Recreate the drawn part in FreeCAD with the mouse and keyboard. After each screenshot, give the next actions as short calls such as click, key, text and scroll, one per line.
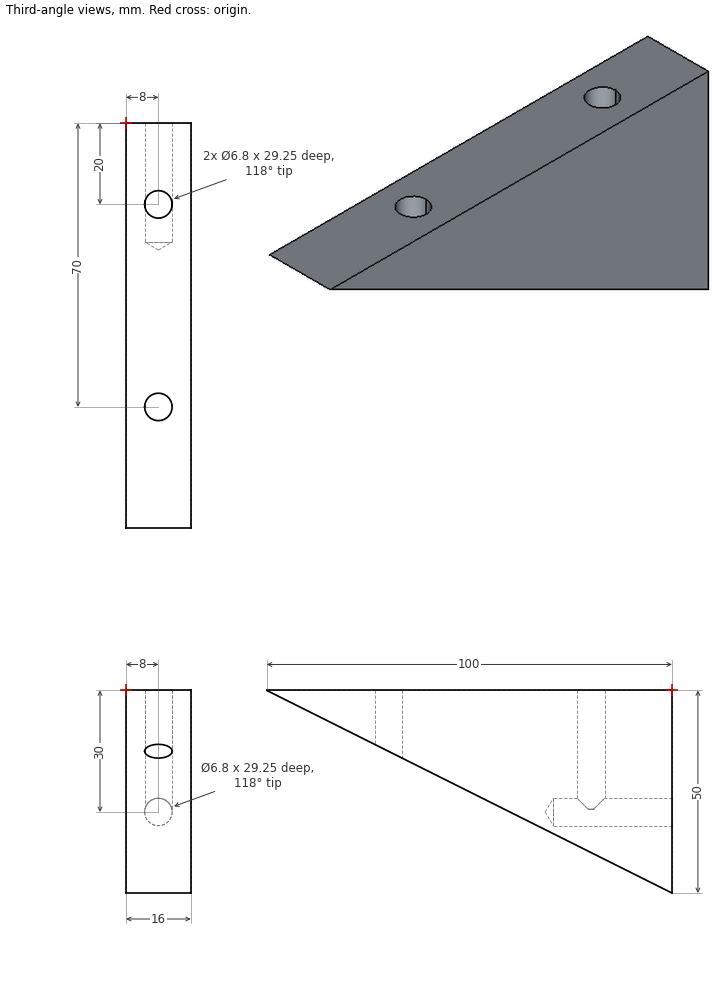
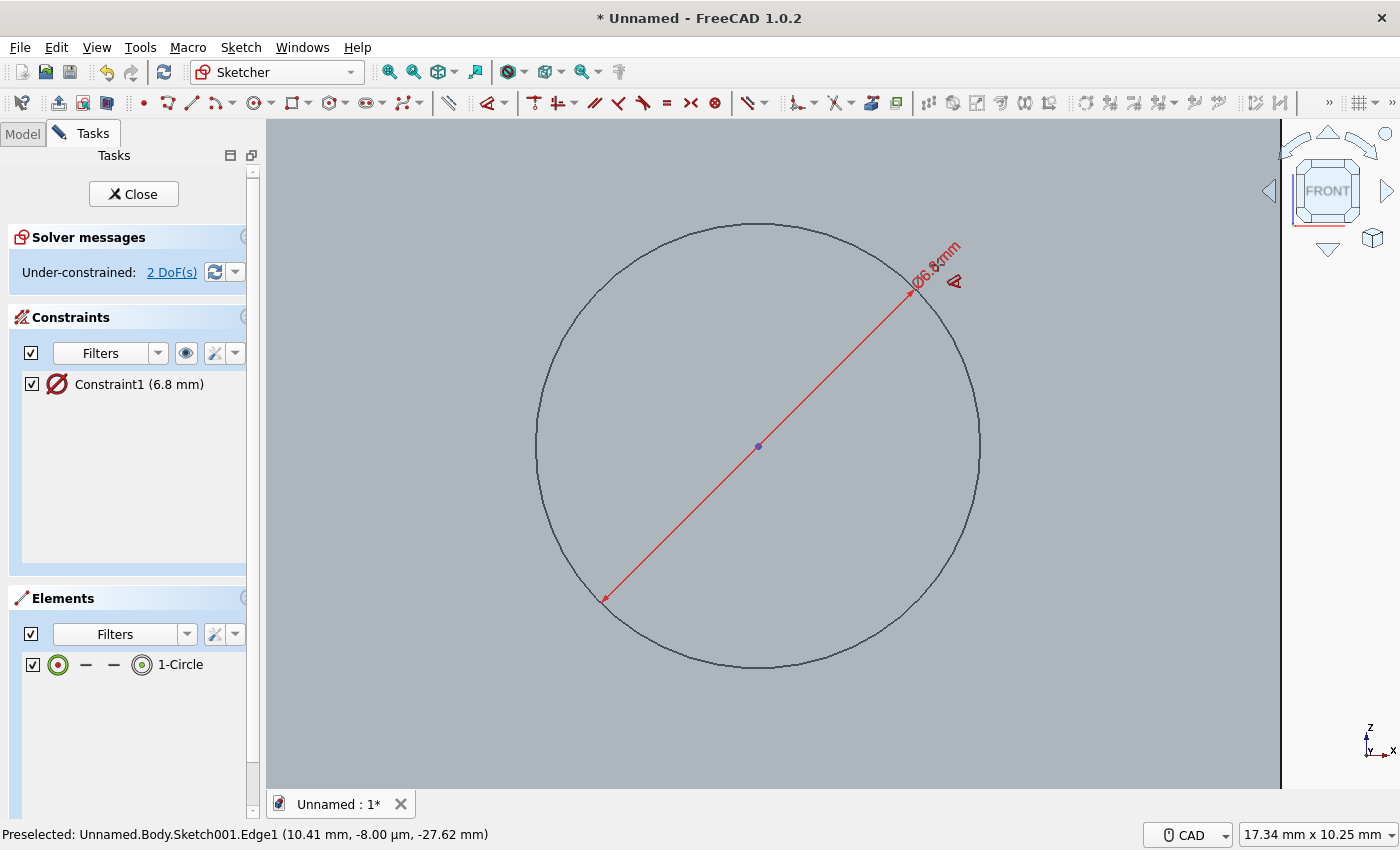
click(758, 446)
click(419, 480)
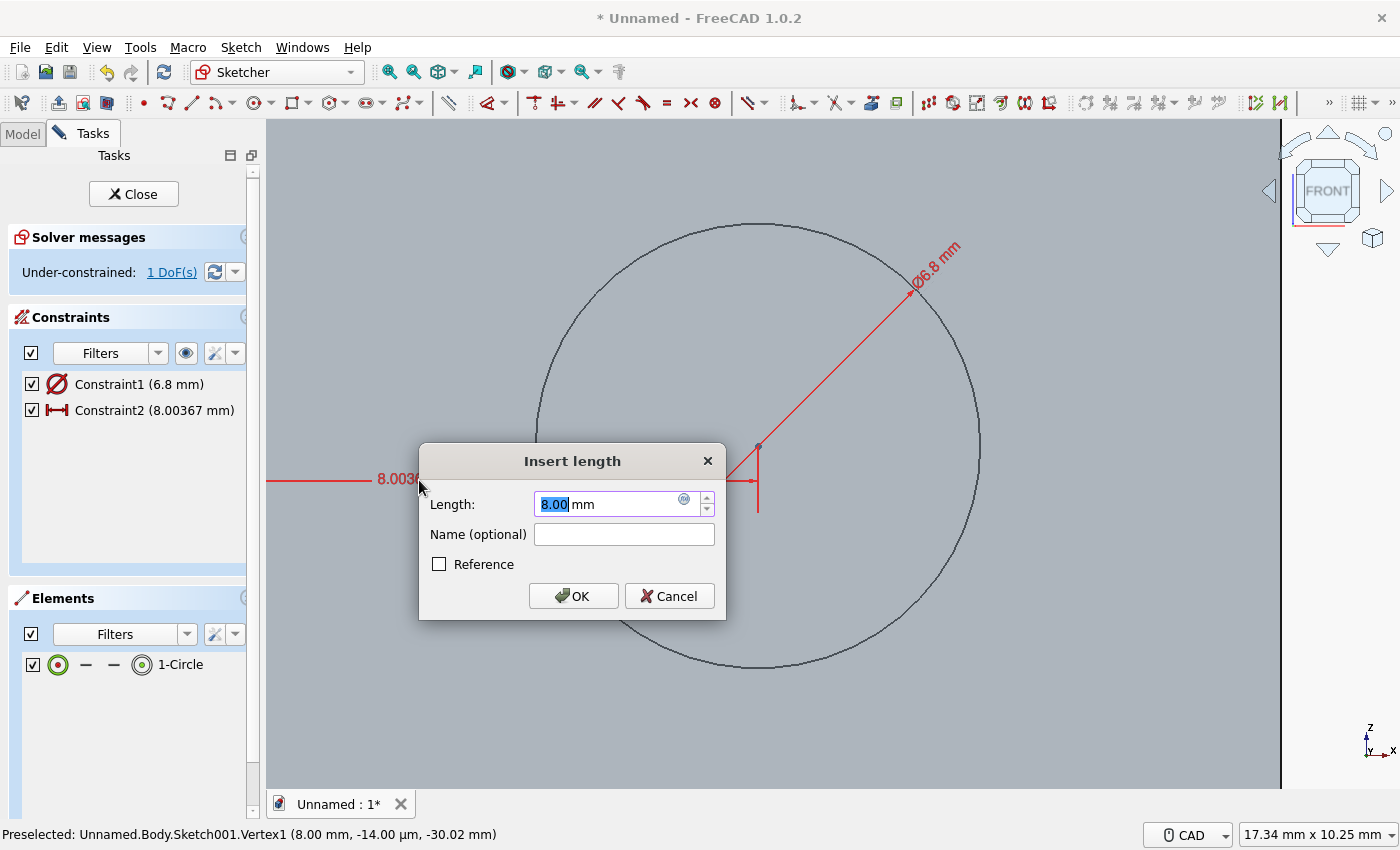
text(8)
key(Return)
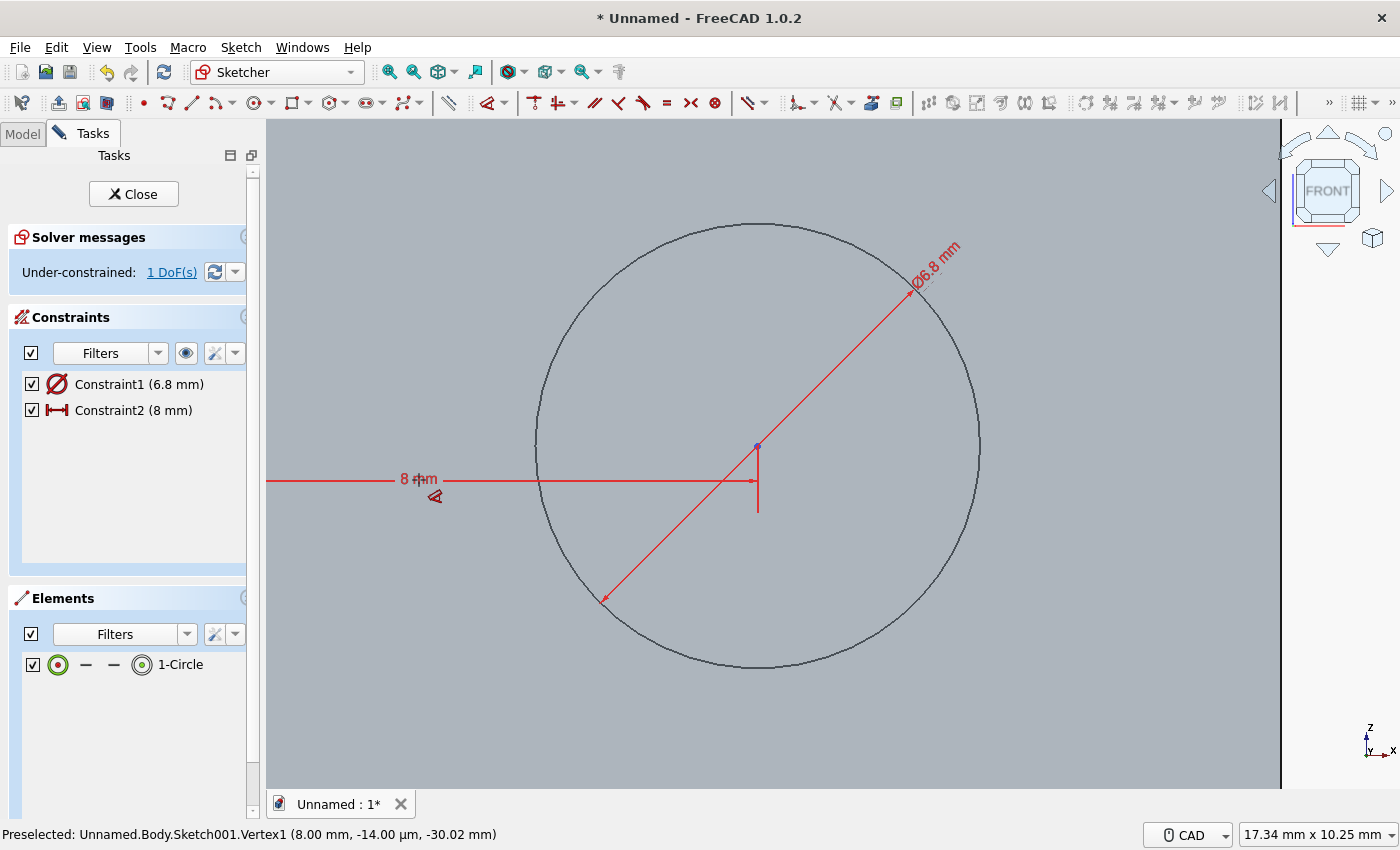
click(758, 446)
click(792, 297)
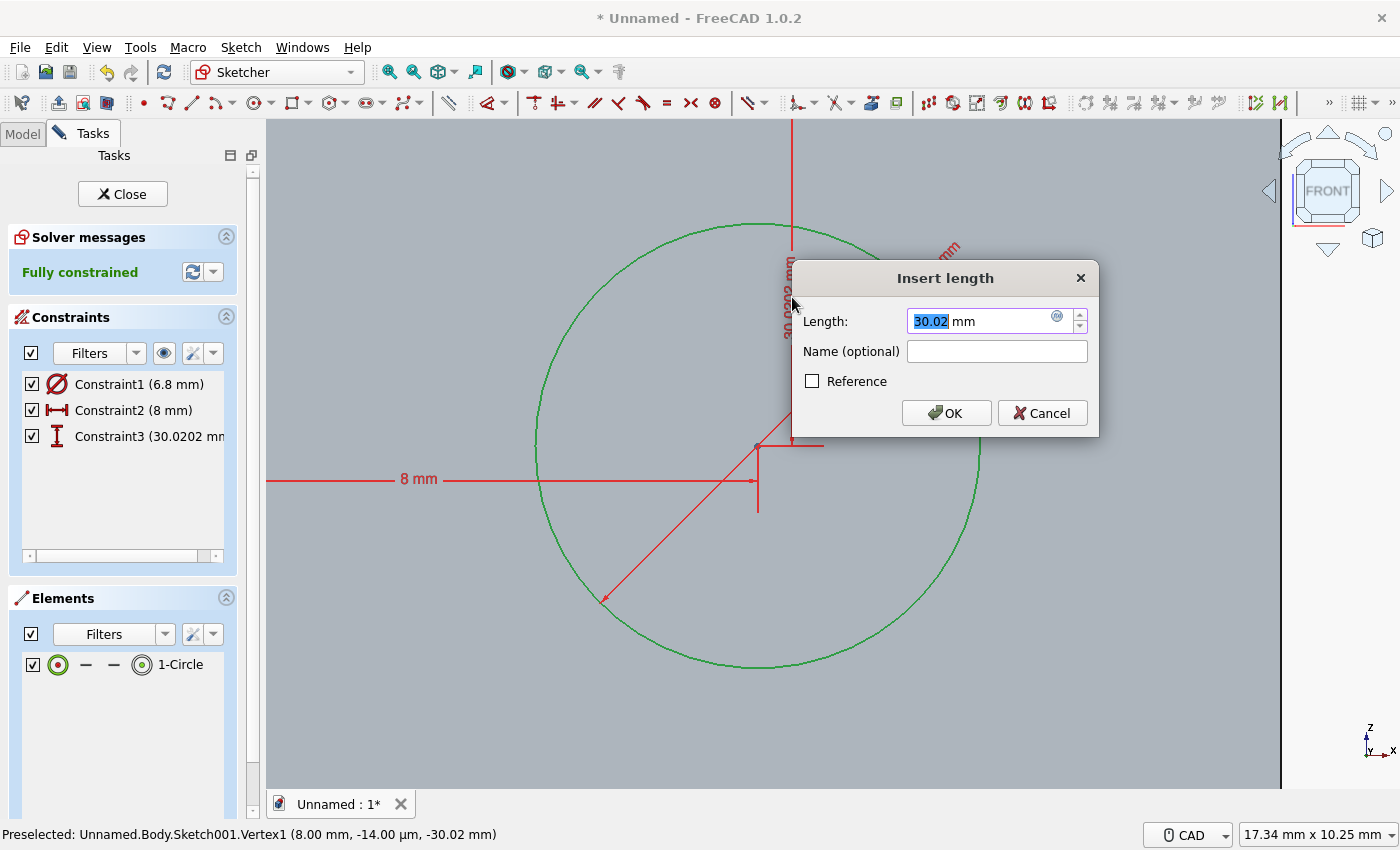
text(30)
key(Return)
key(Escape)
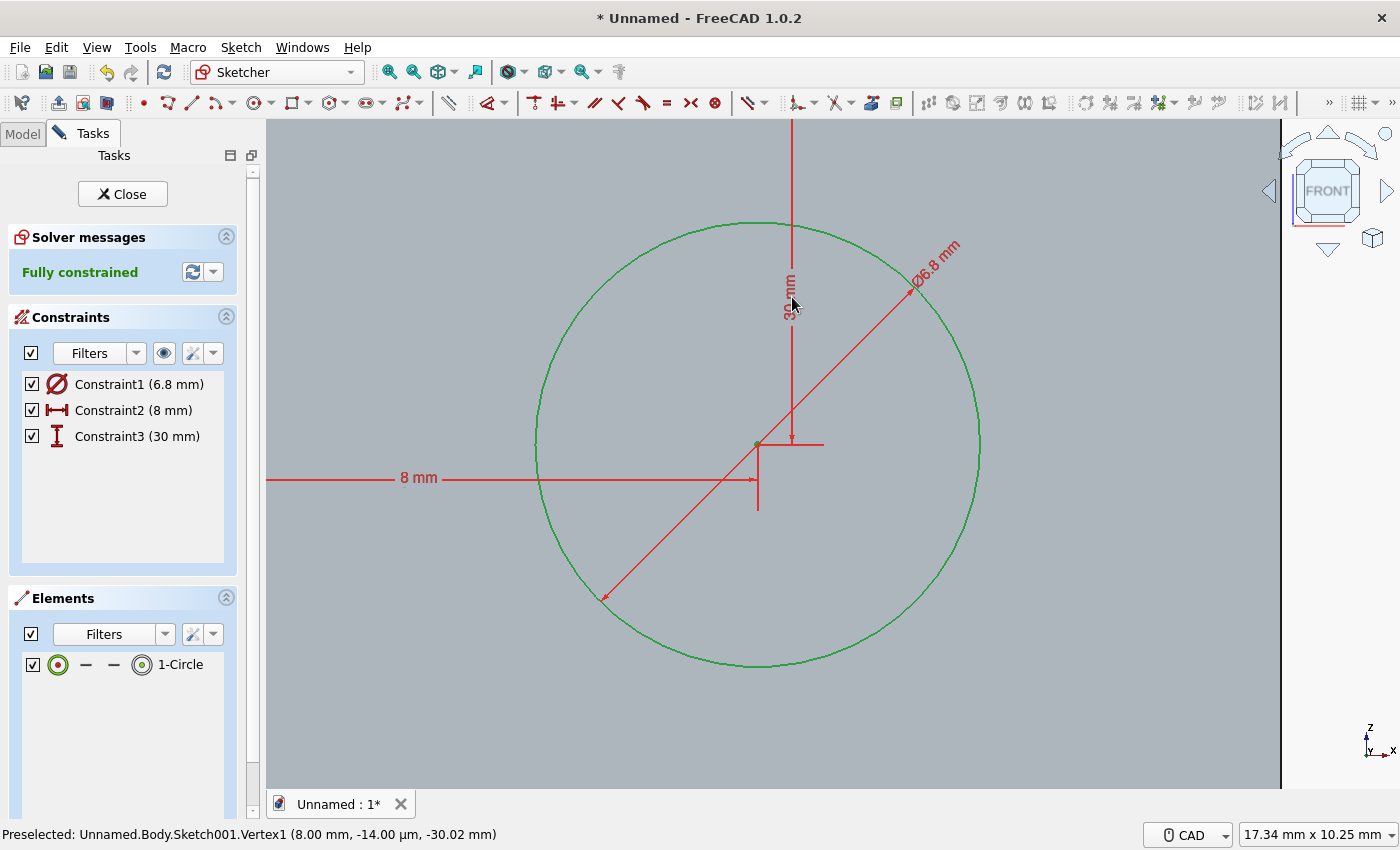
click(123, 194)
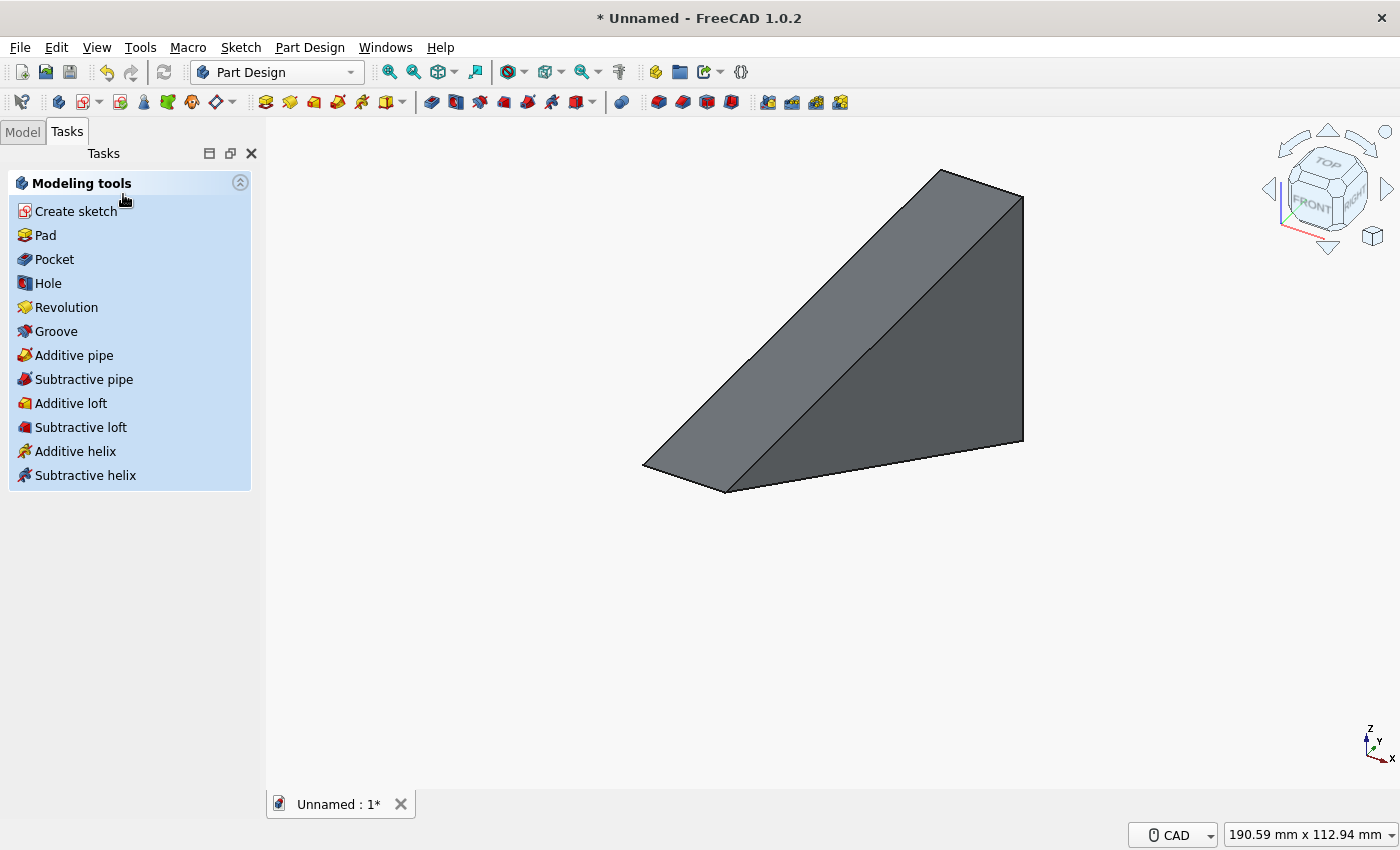
click(456, 102)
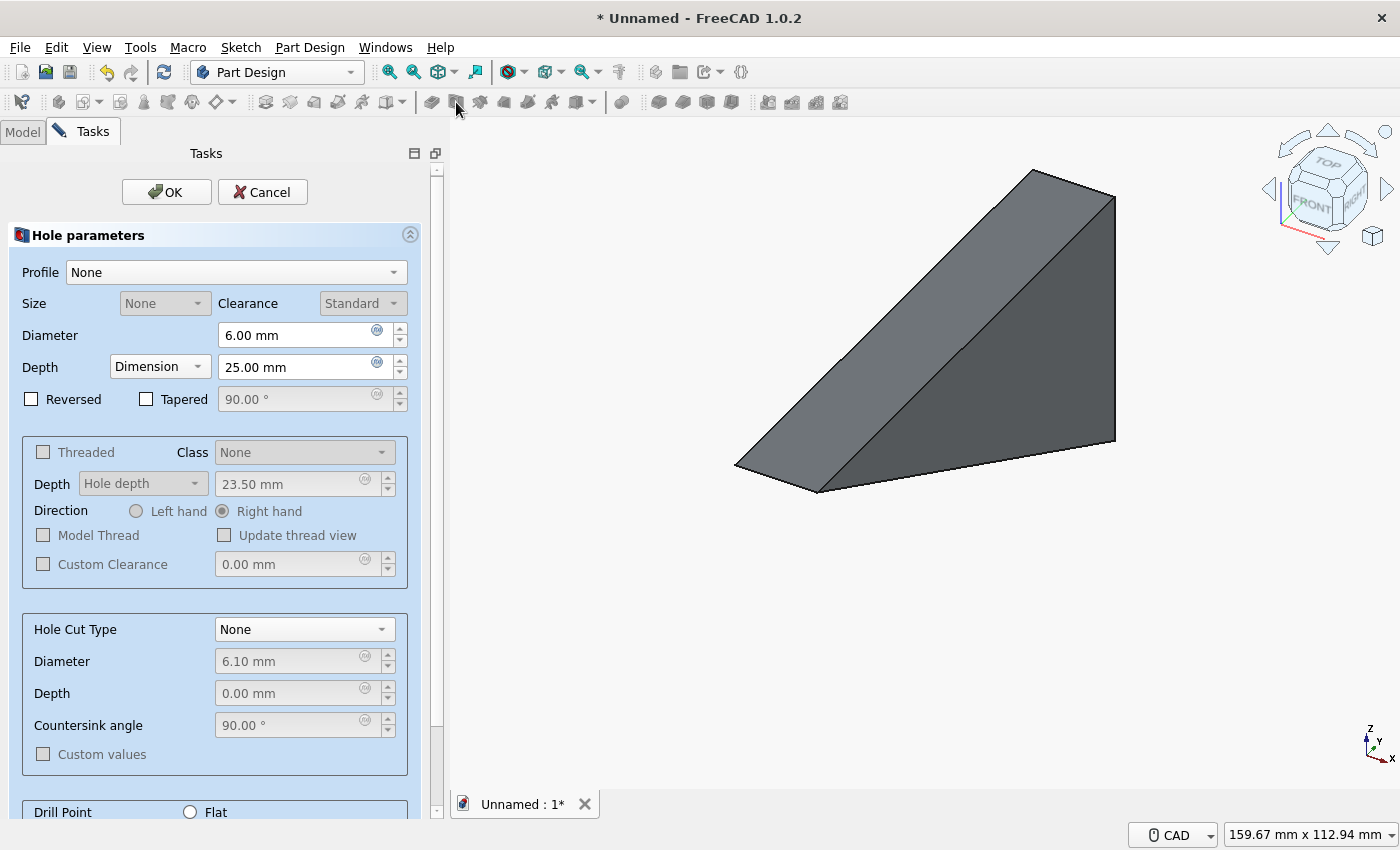
triple_click(305, 335)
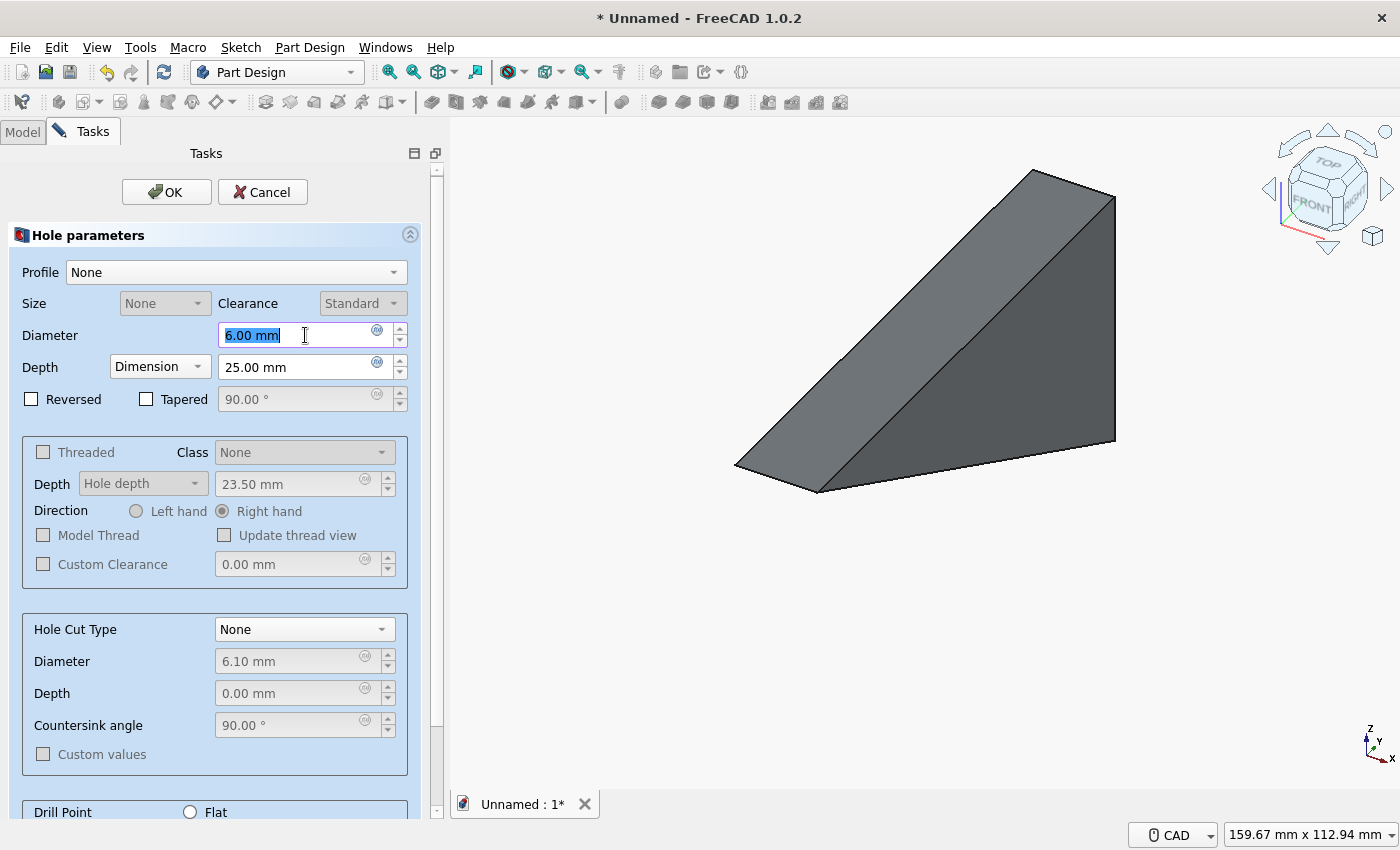
text(6.8)
key(Tab)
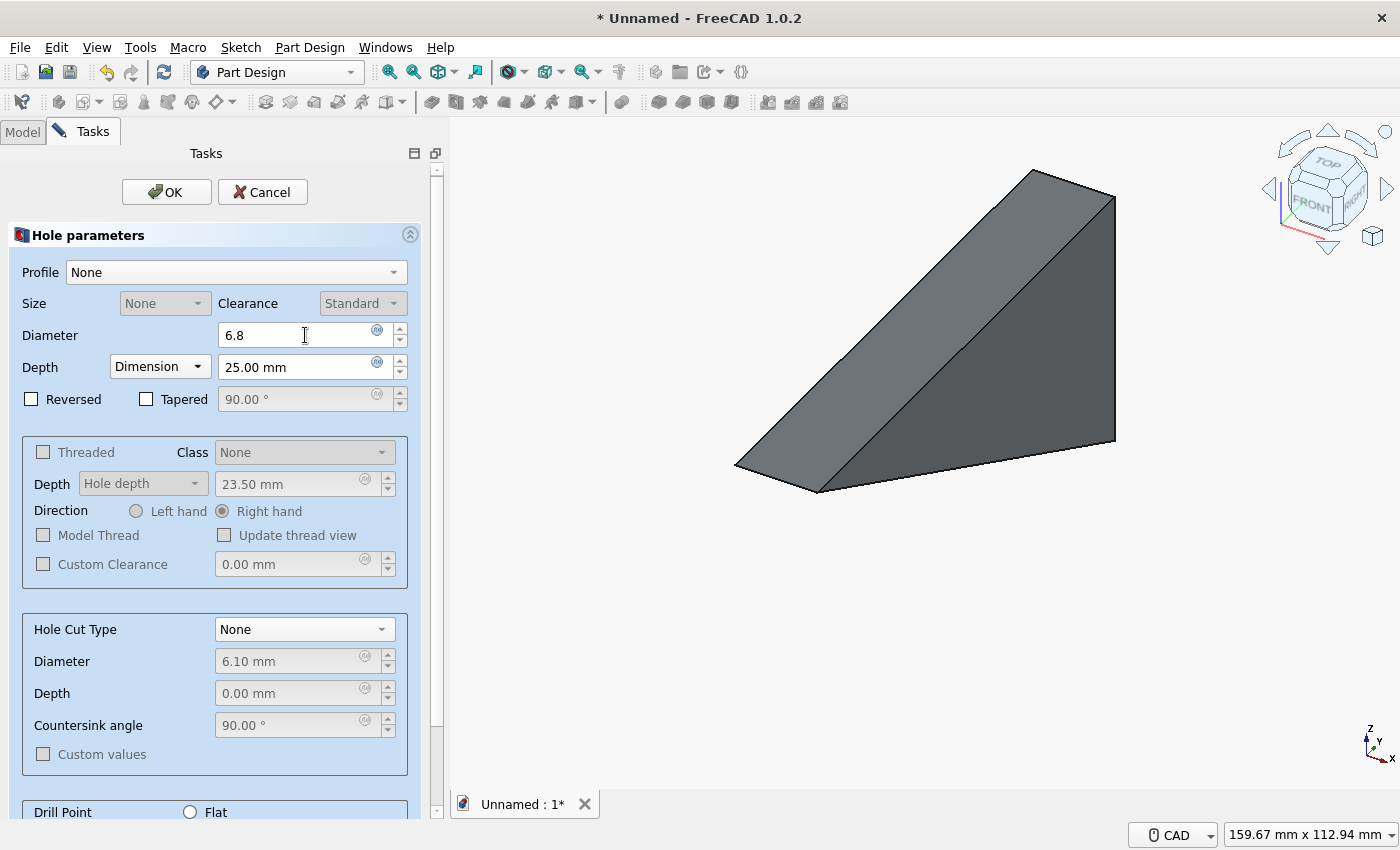
triple_click(305, 367)